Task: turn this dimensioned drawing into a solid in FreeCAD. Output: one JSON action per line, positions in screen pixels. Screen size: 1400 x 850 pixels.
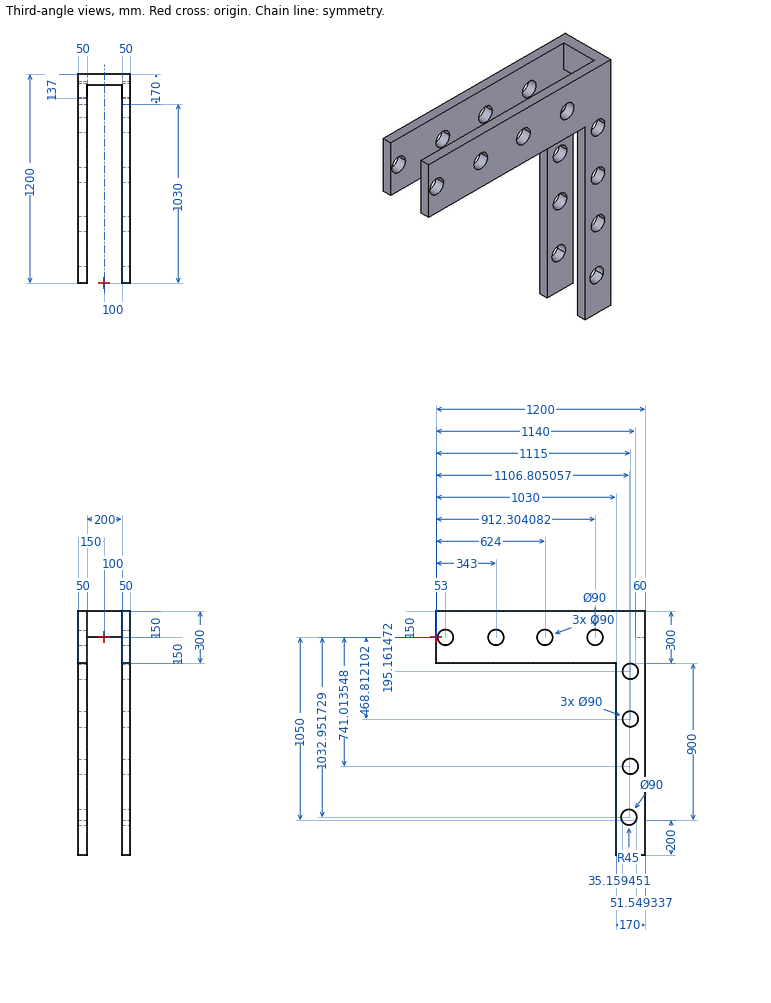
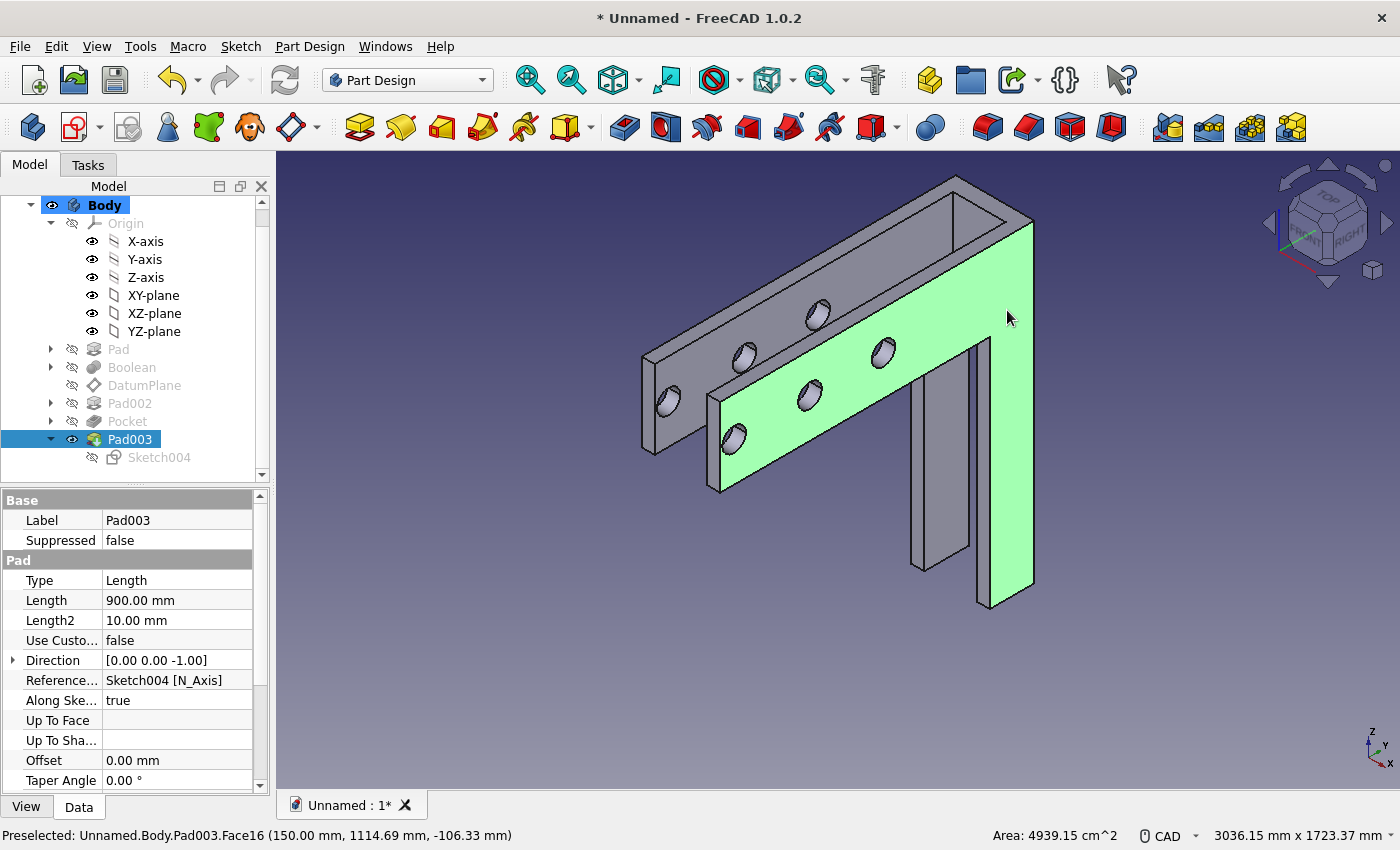
{"action": "left_click", "coordinate": [74, 128]}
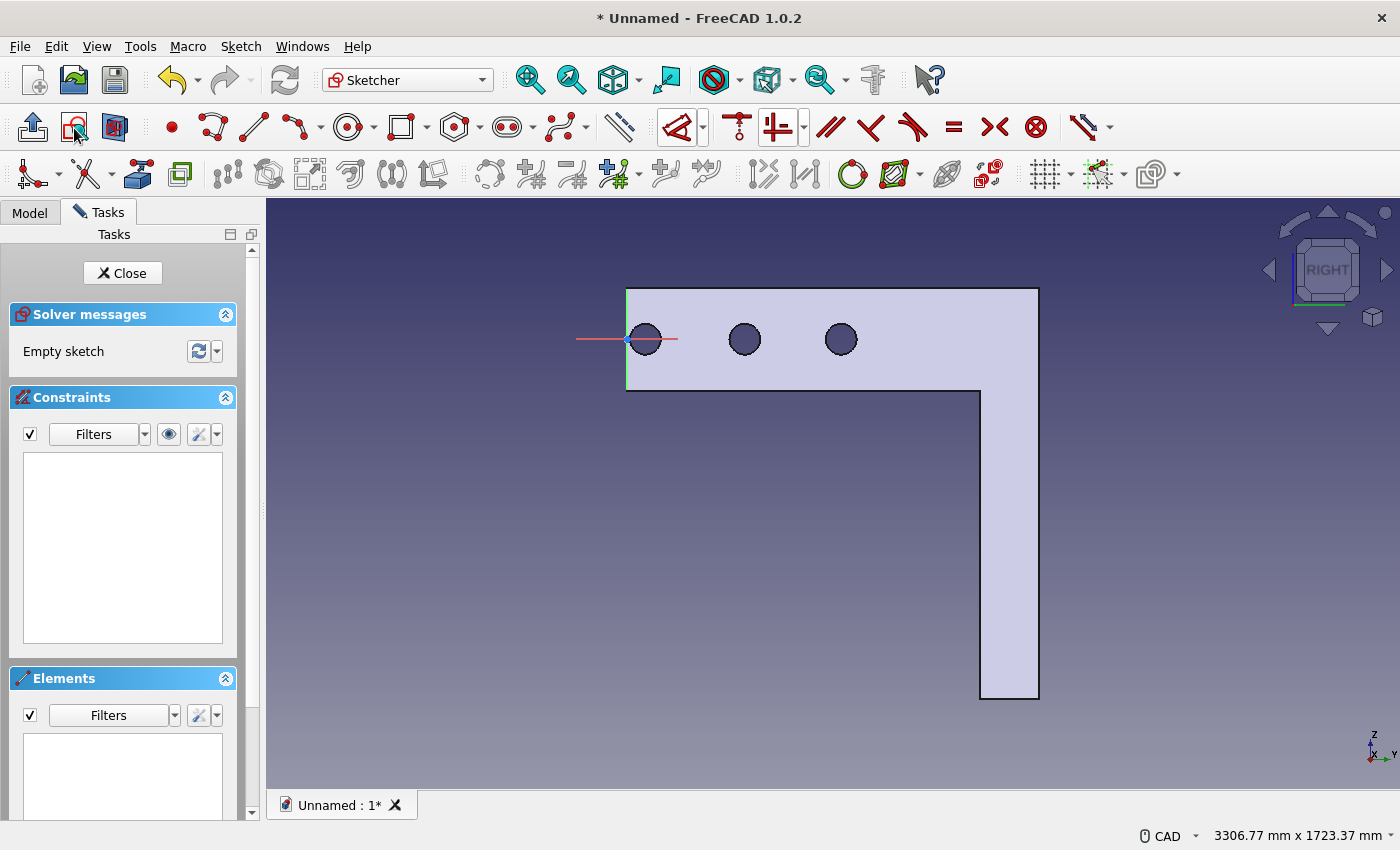
{"action": "scroll", "coordinate": [951, 434], "scroll_direction": "up", "scroll_amount": 2}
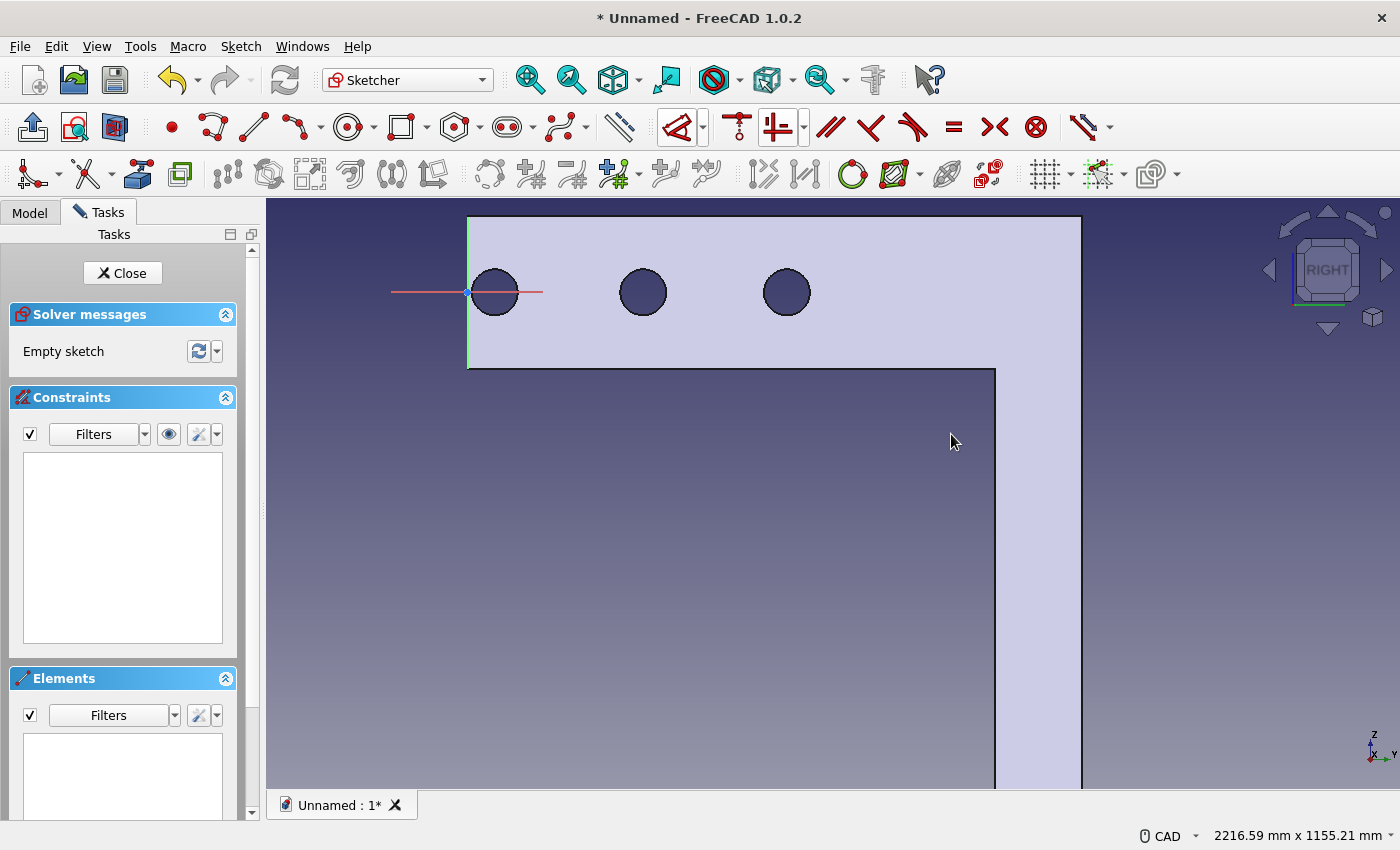
{"action": "left_click", "coordinate": [348, 128]}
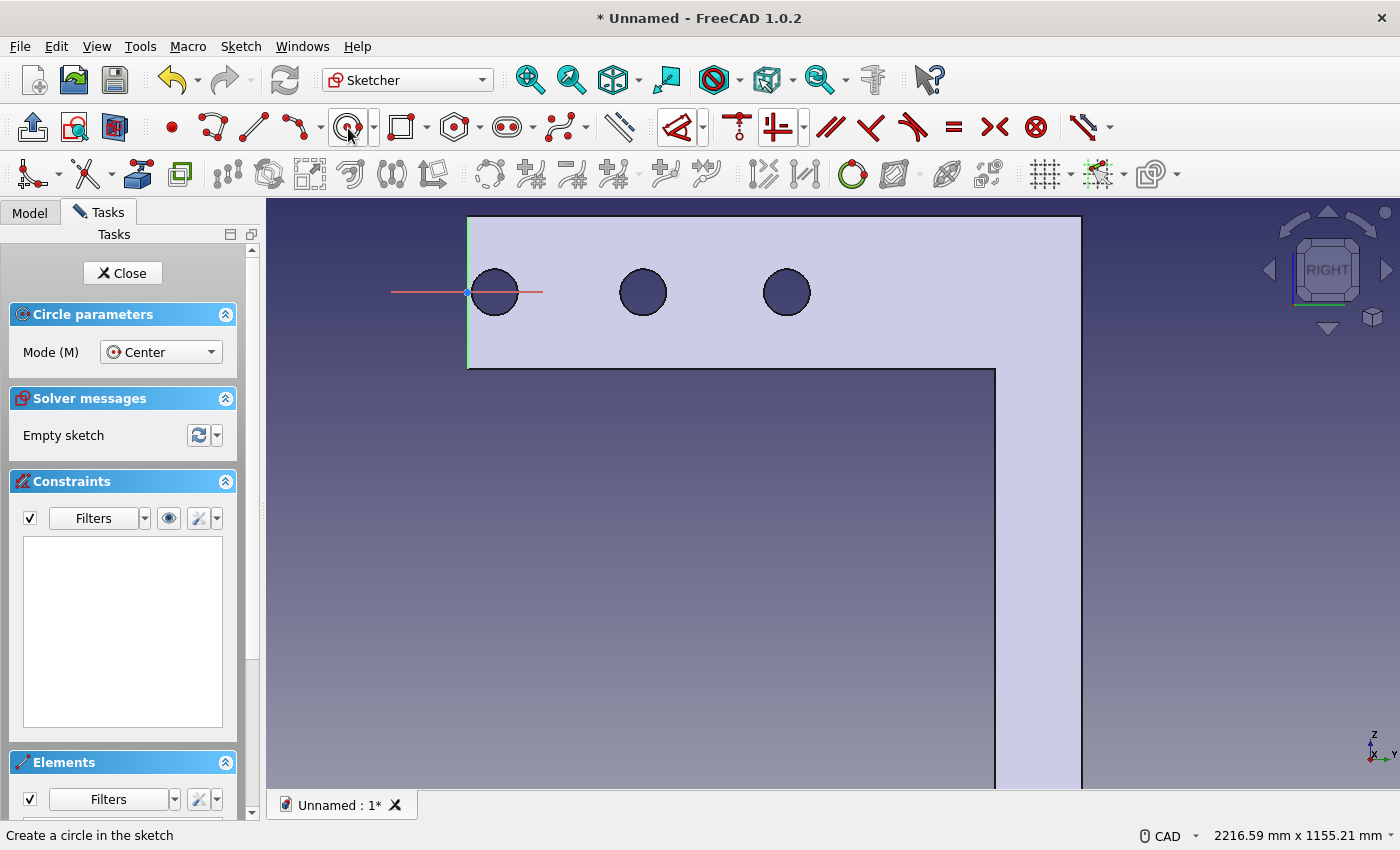
{"action": "left_click", "coordinate": [1038, 532]}
{"action": "left_click", "coordinate": [1054, 516]}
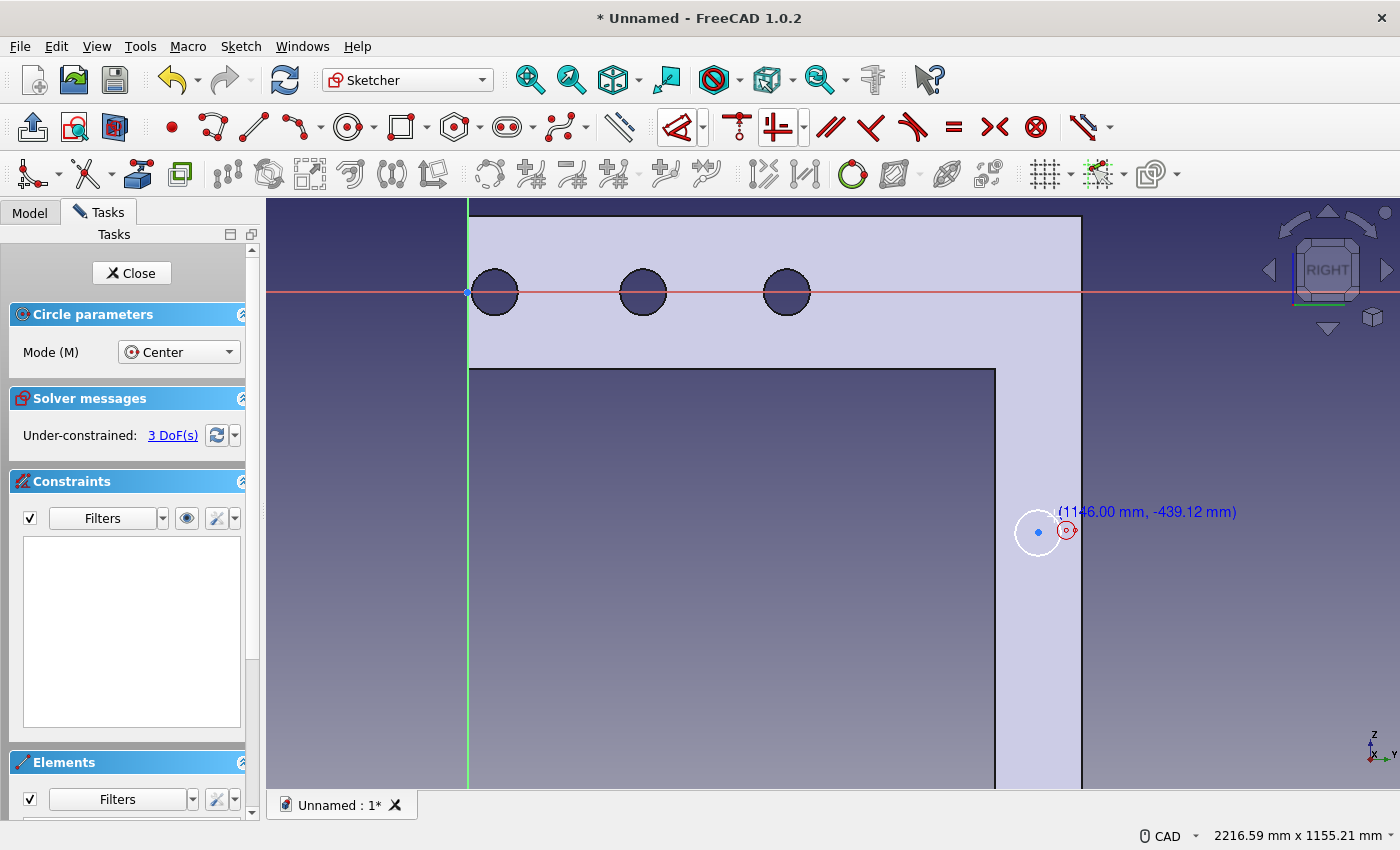
{"action": "left_click", "coordinate": [1038, 671]}
{"action": "left_click", "coordinate": [1054, 655]}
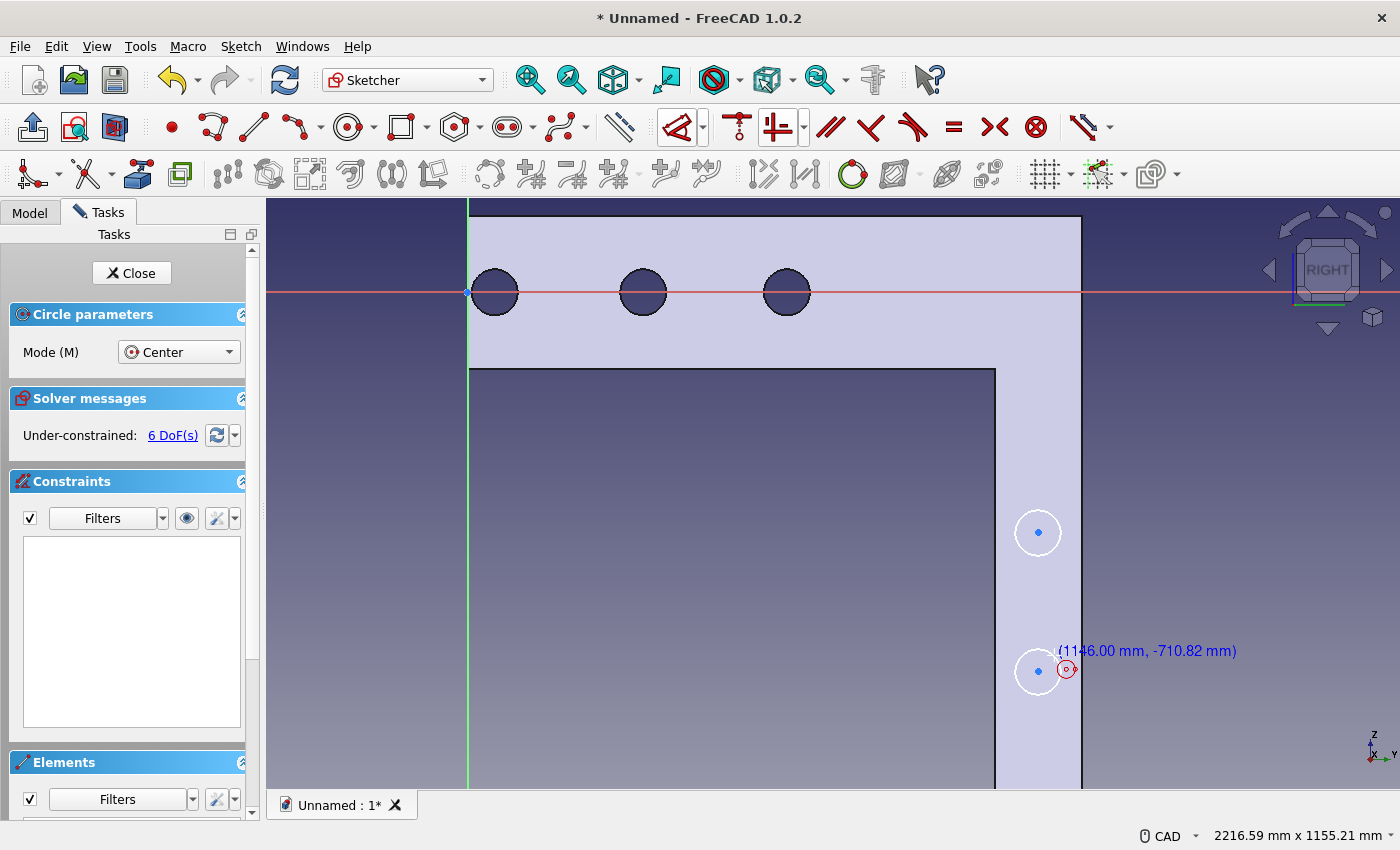
{"action": "left_click", "coordinate": [1038, 392]}
{"action": "left_click", "coordinate": [1054, 376]}
{"action": "key", "text": "Escape"}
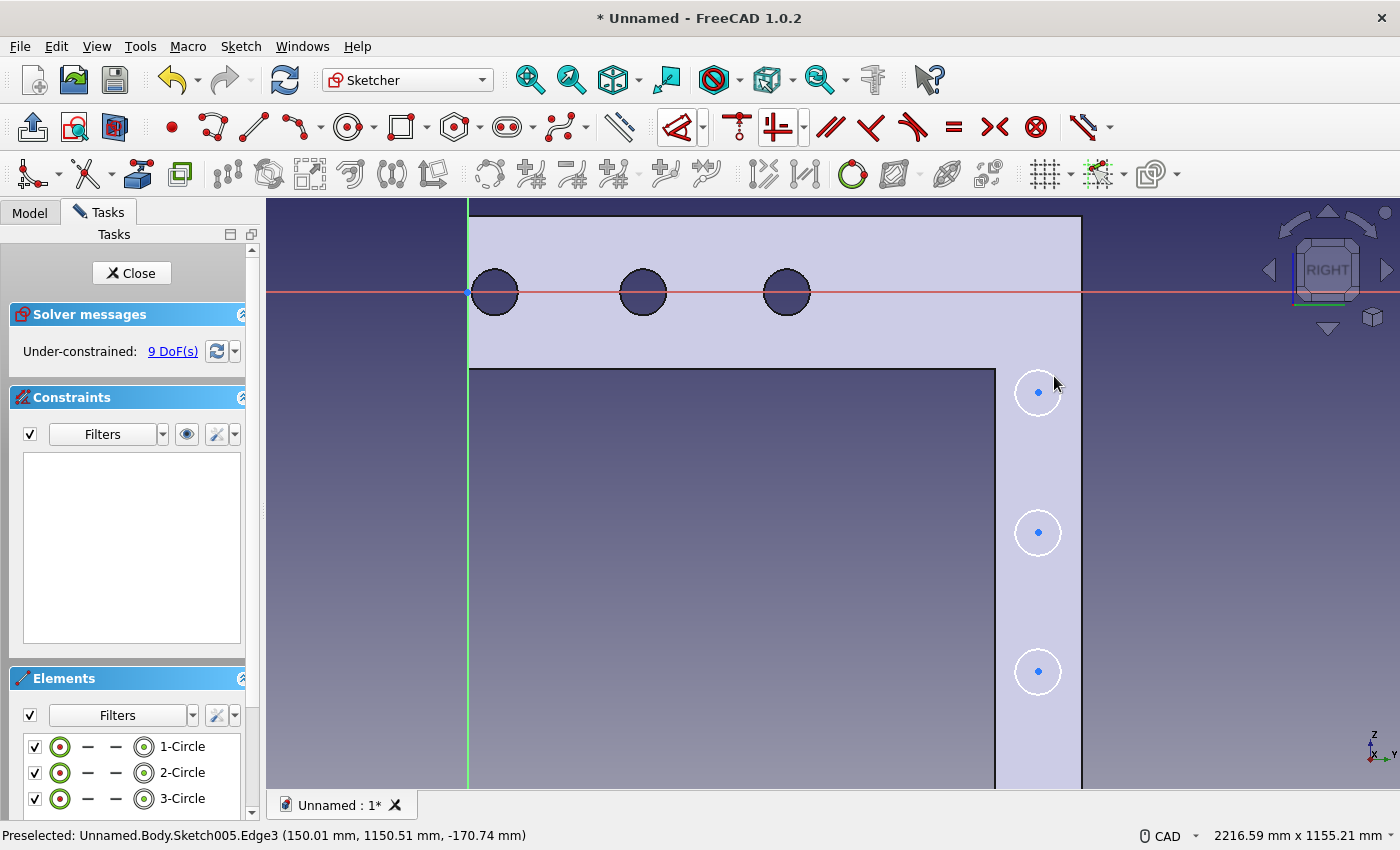
{"action": "left_click", "coordinate": [1054, 517]}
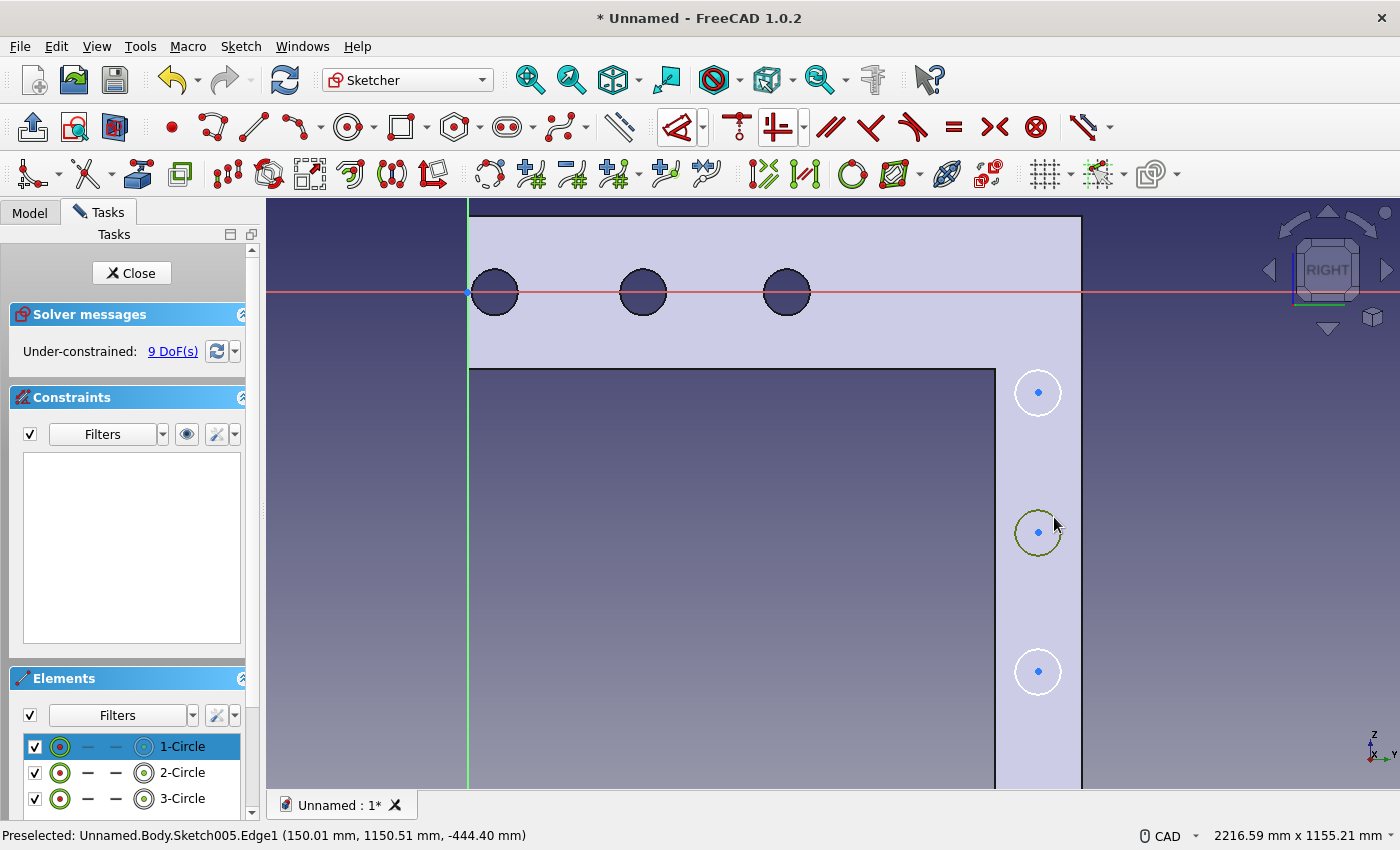
{"action": "left_click", "coordinate": [1054, 656]}